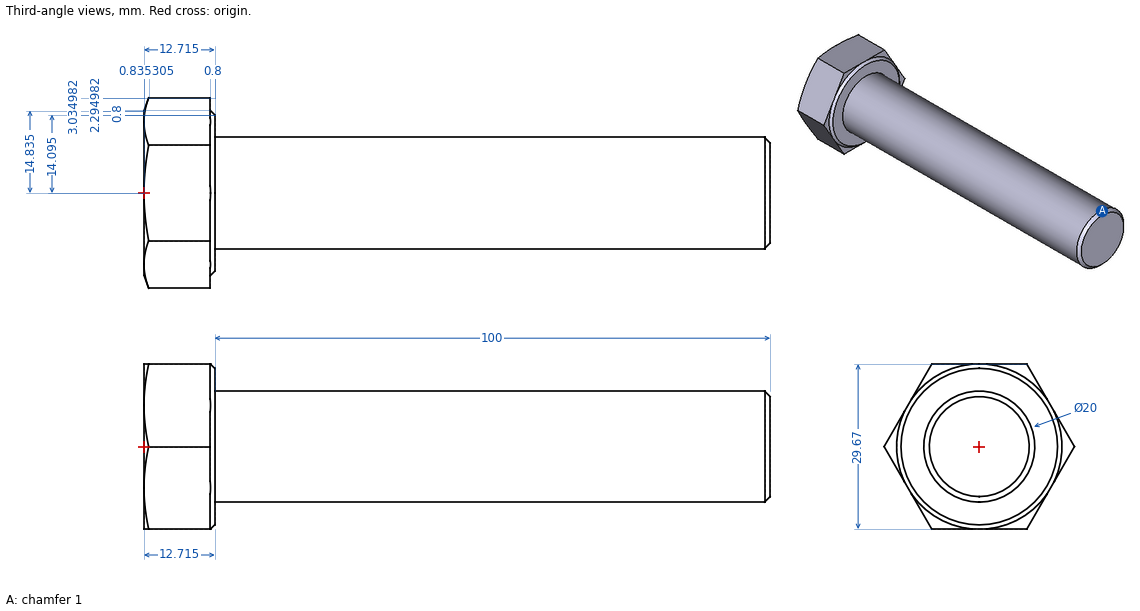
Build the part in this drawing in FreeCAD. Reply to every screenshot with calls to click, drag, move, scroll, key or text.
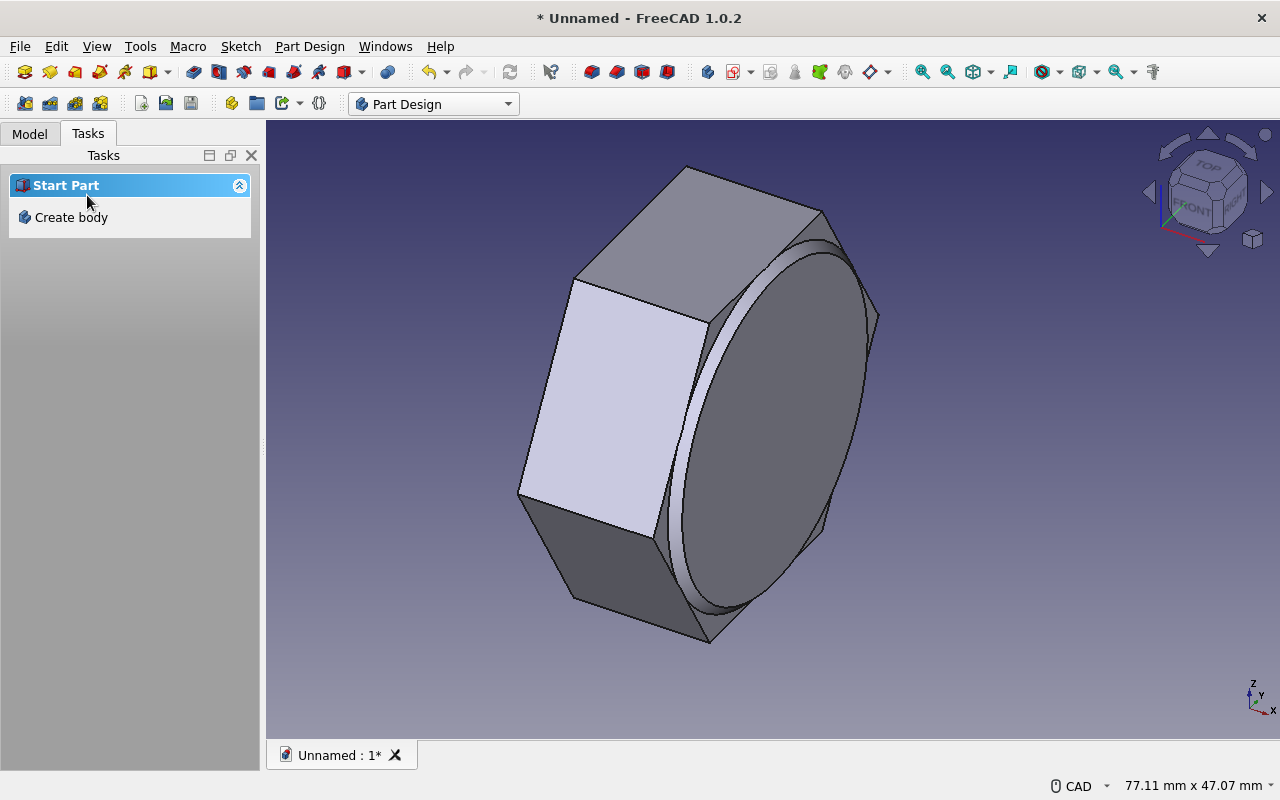
key(v)
key(f)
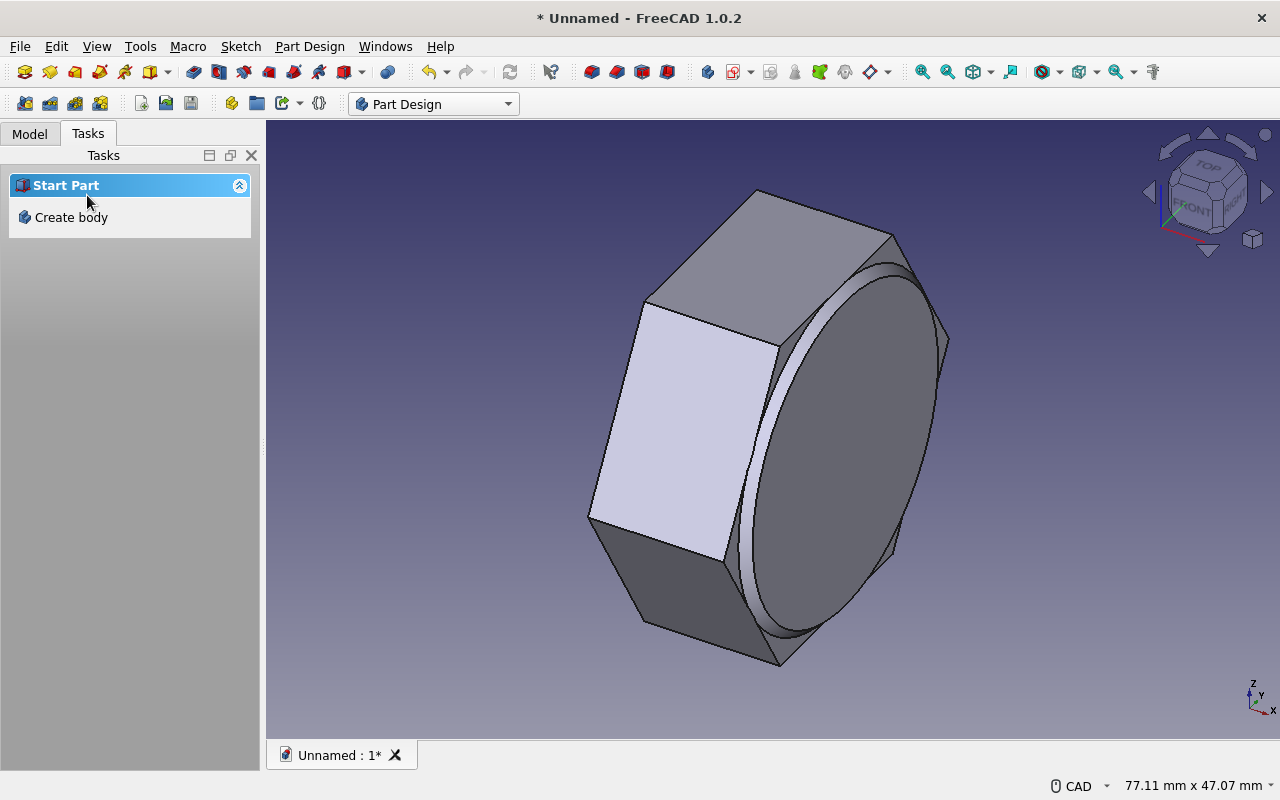
click(732, 72)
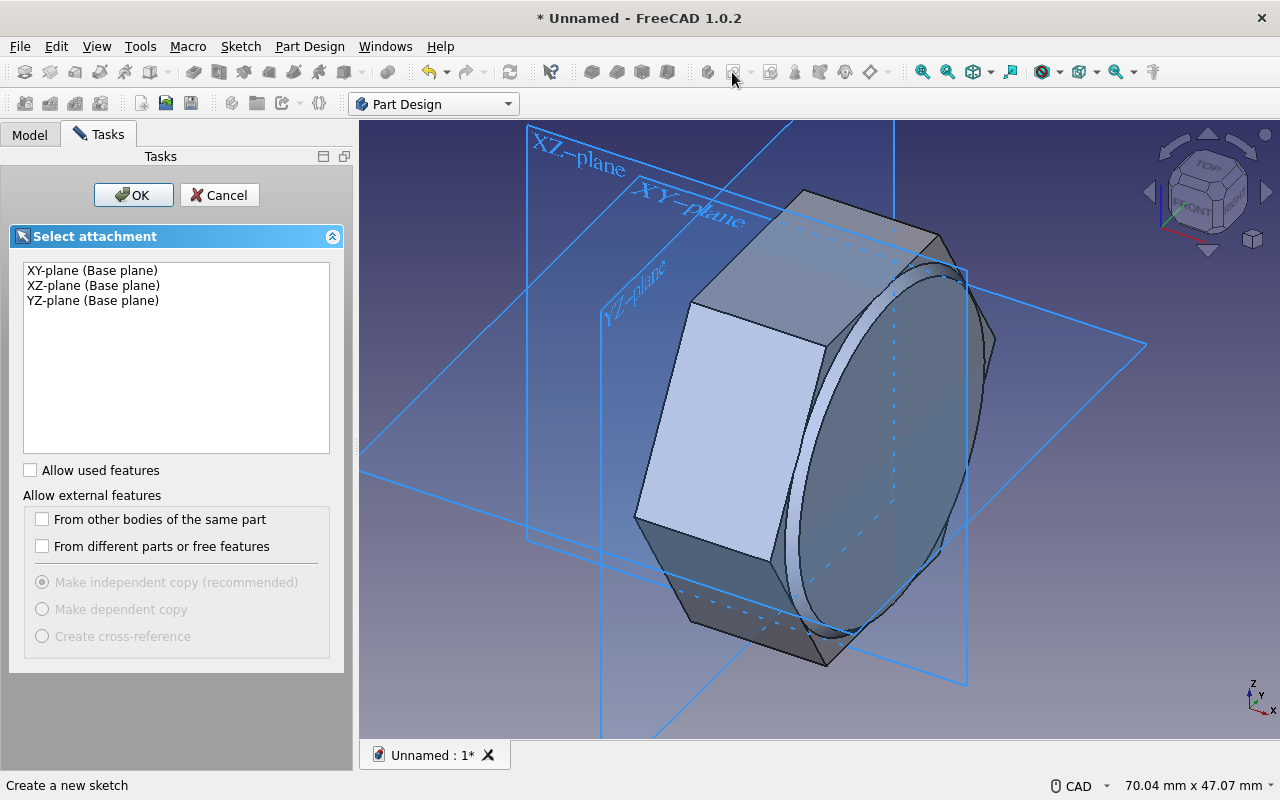
click(84, 270)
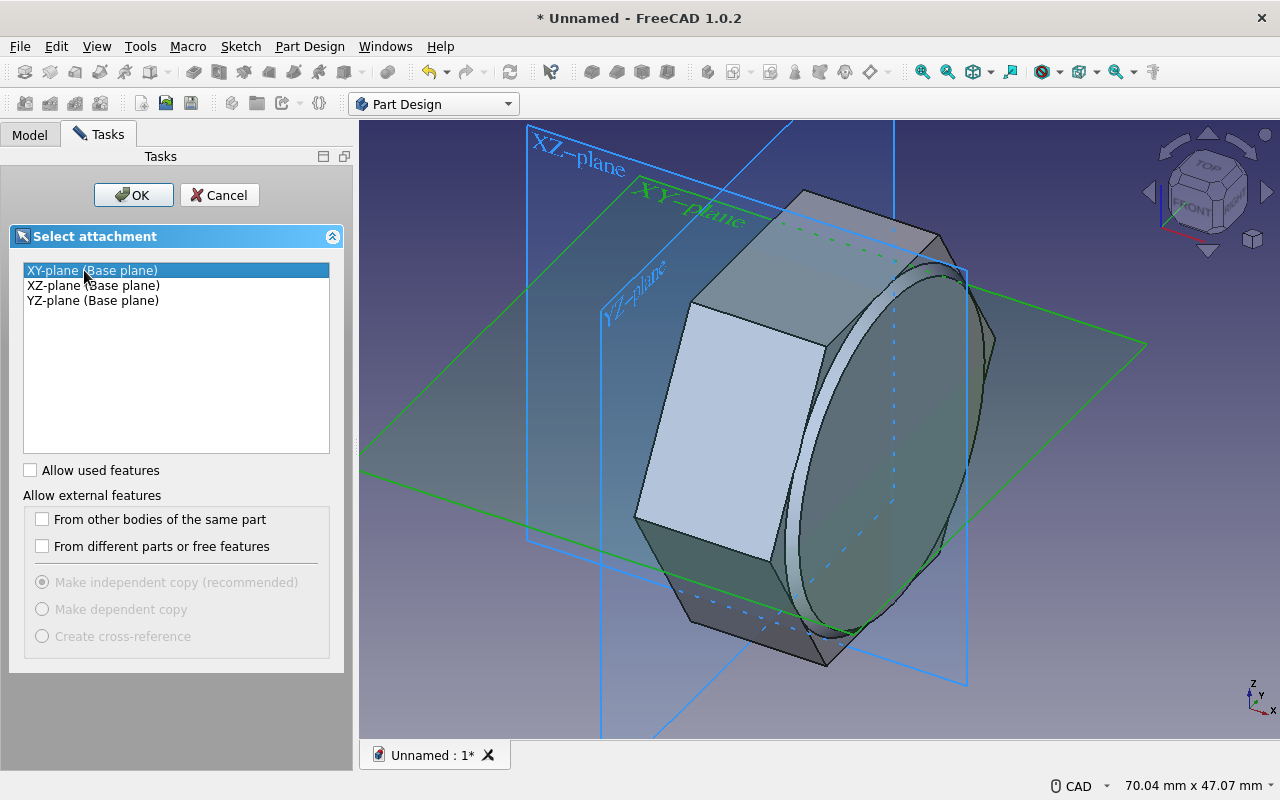
click(134, 195)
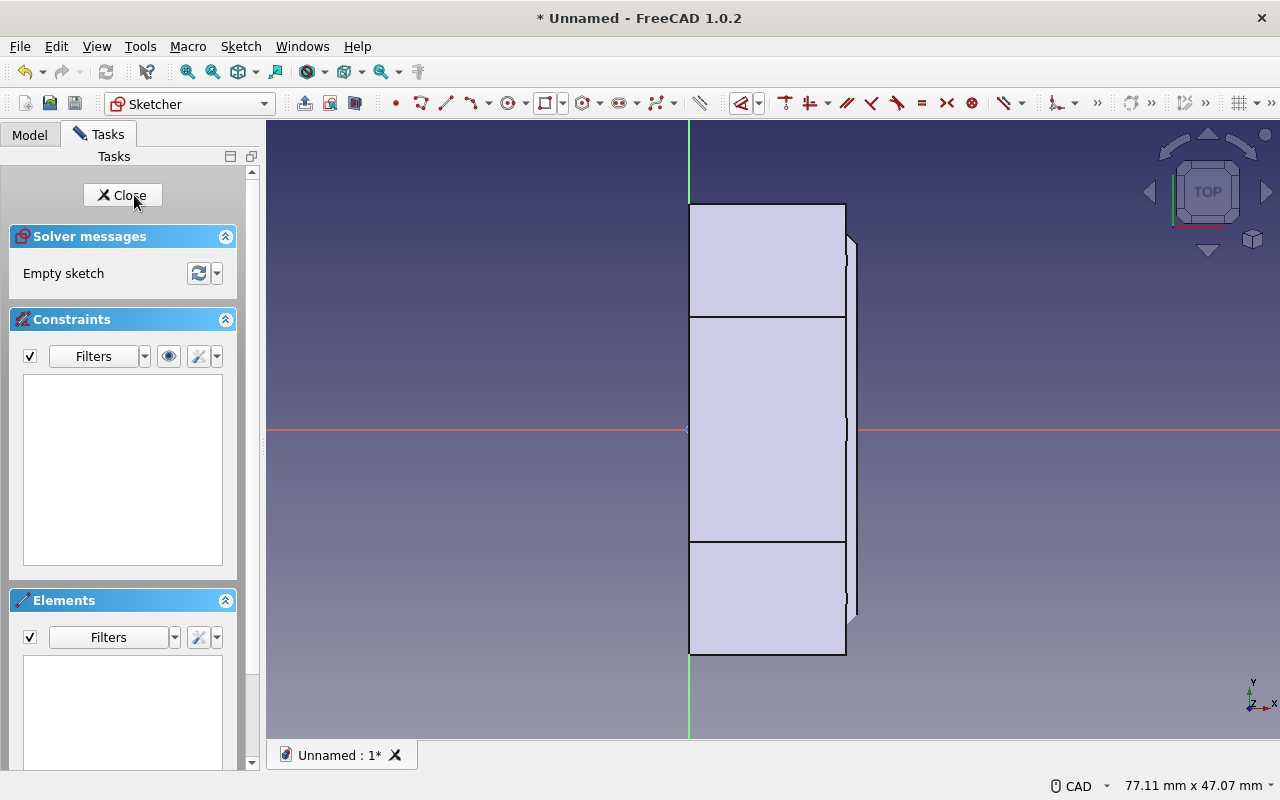
key(q)
key(s)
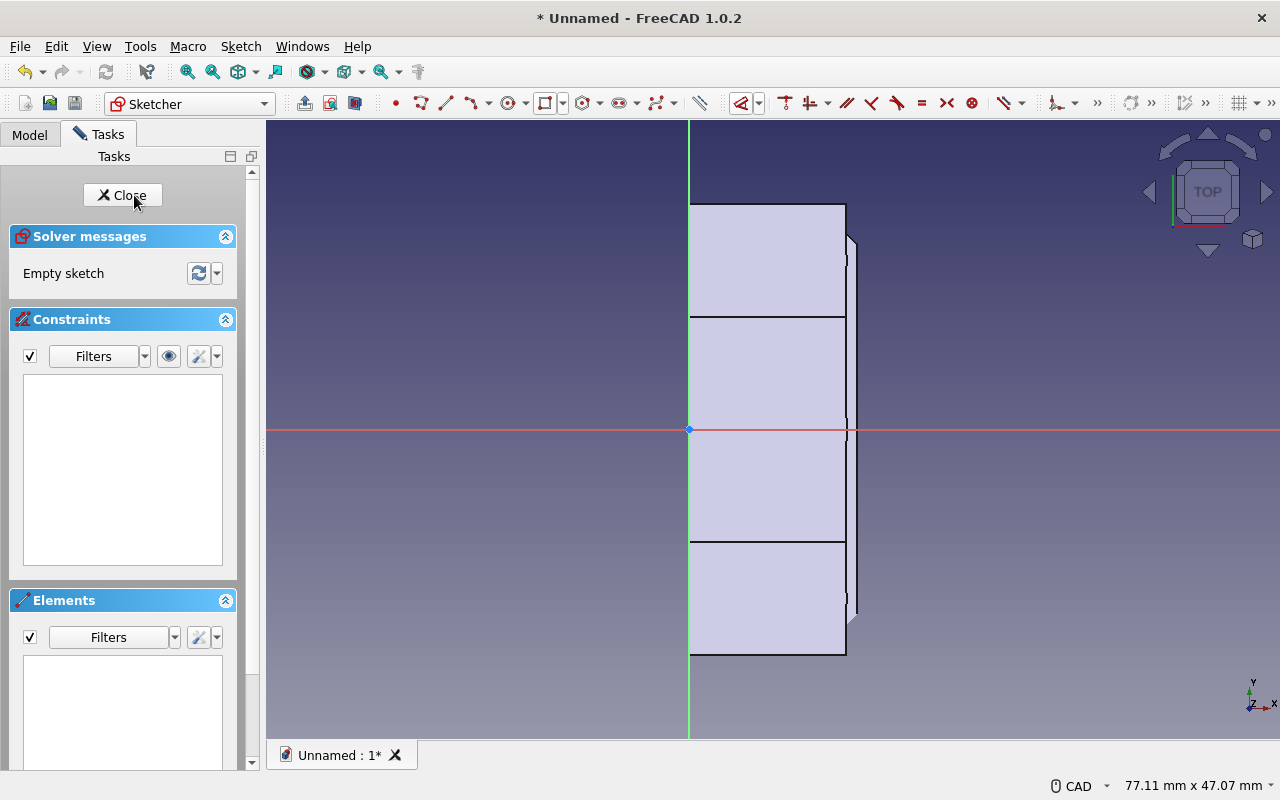
scroll(694, 202, up, 13)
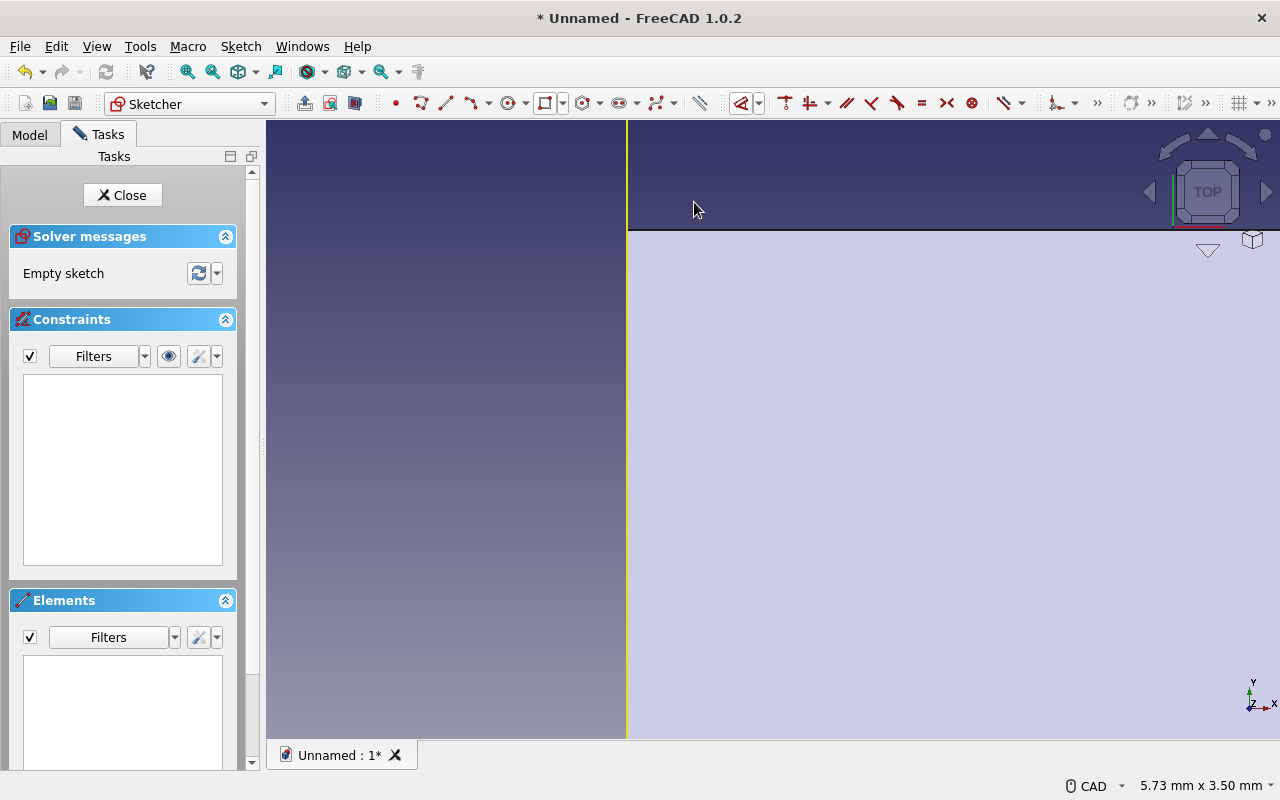
key(g)
key(m)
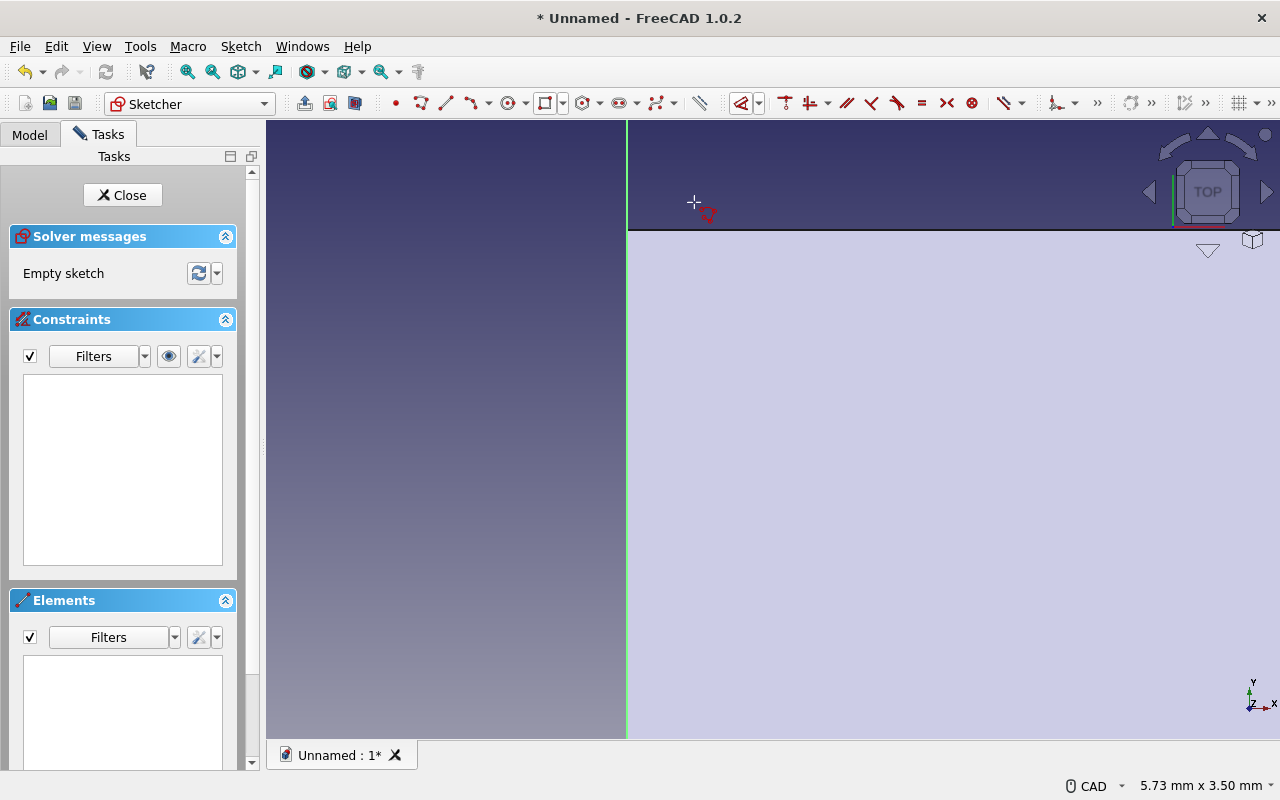
click(627, 637)
click(775, 230)
click(636, 230)
click(627, 638)
key(Escape)
key(Escape)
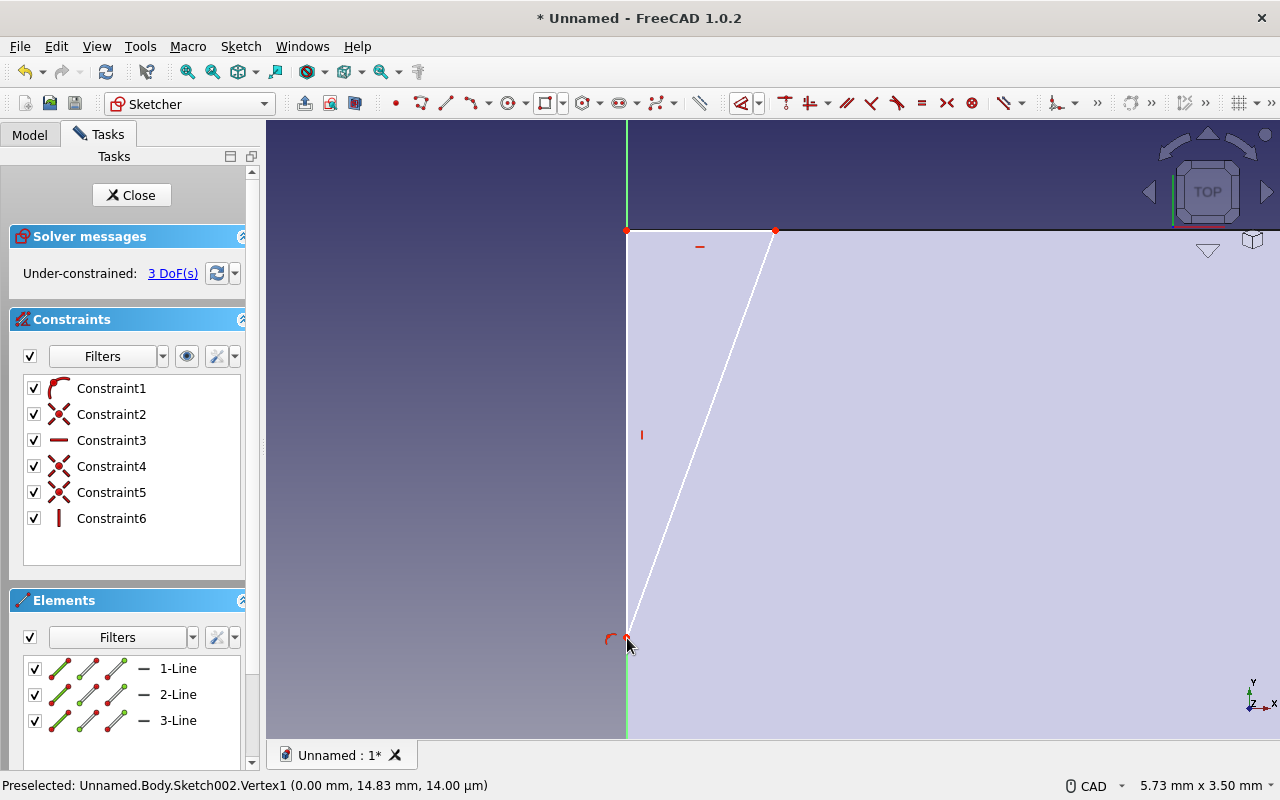
key(d)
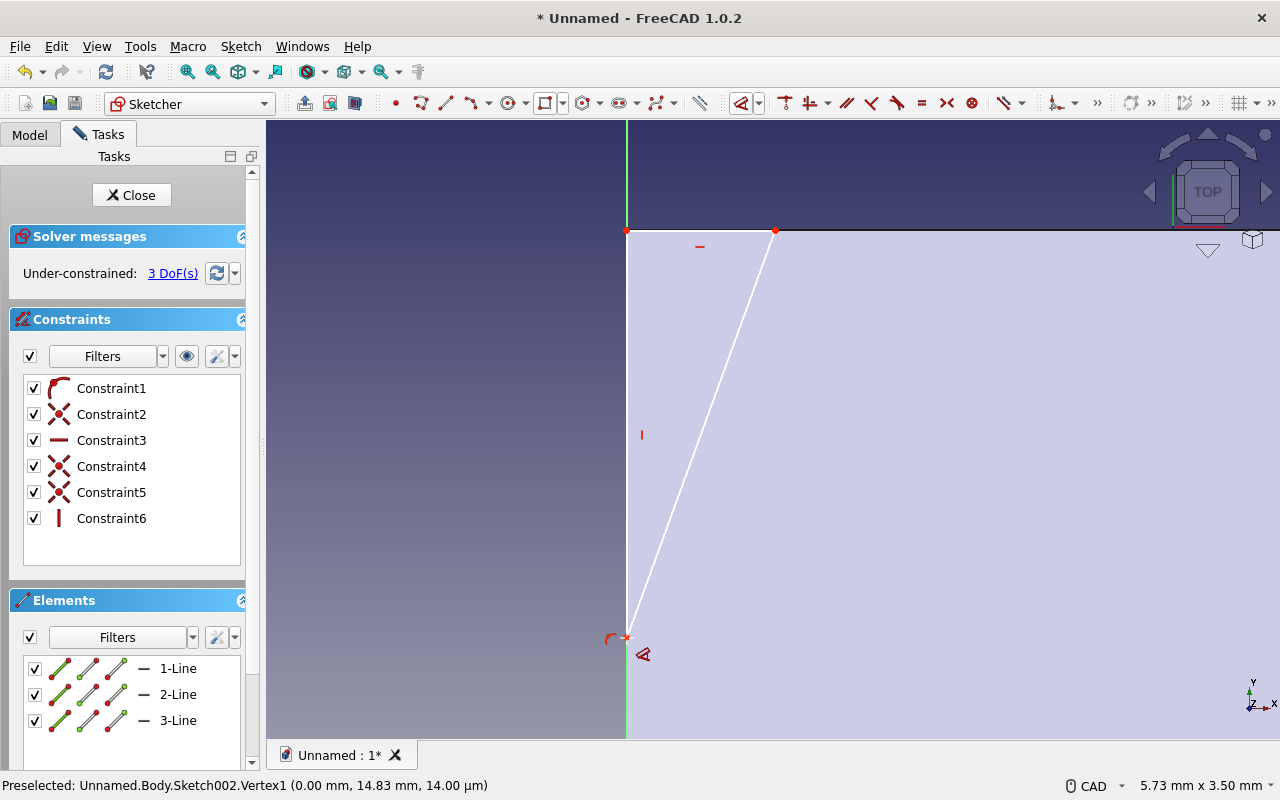
click(627, 638)
click(593, 674)